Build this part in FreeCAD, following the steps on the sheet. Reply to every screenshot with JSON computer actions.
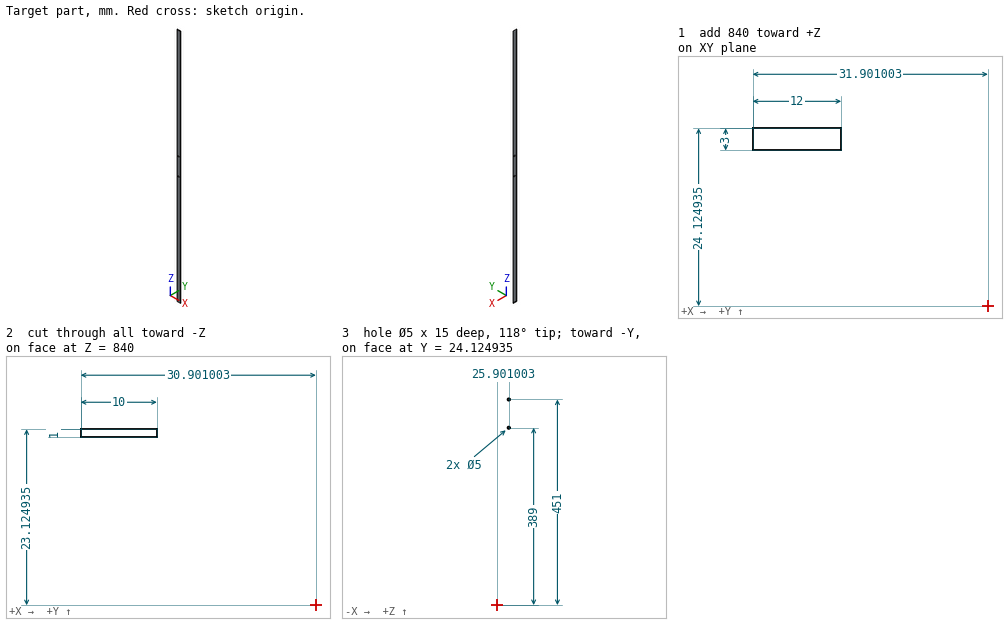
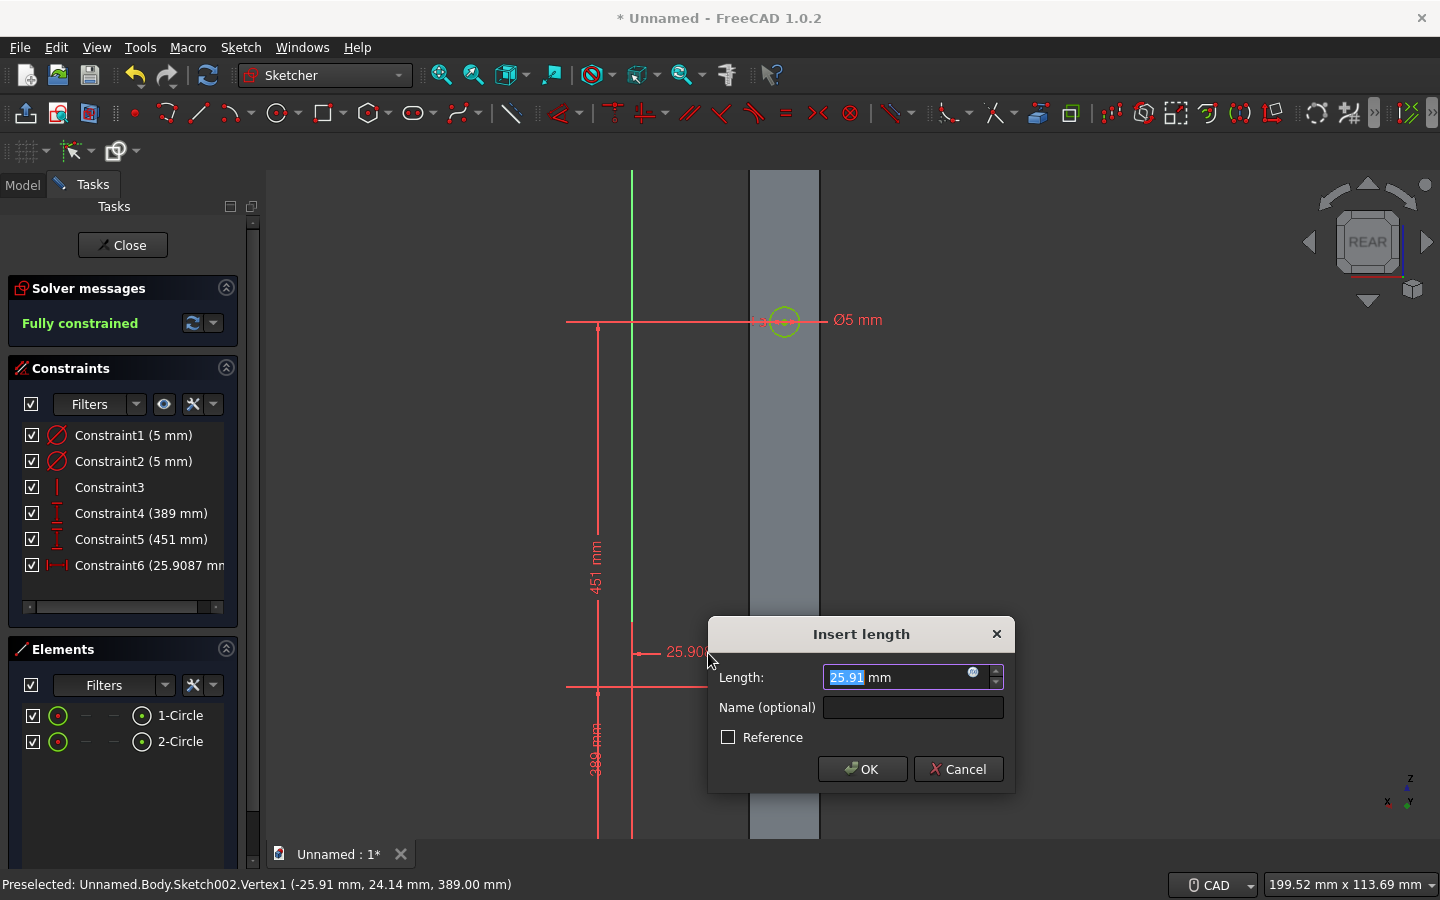
{"action": "type", "text": "25.901003"}
{"action": "key", "text": "Return"}
{"action": "key", "text": "Escape"}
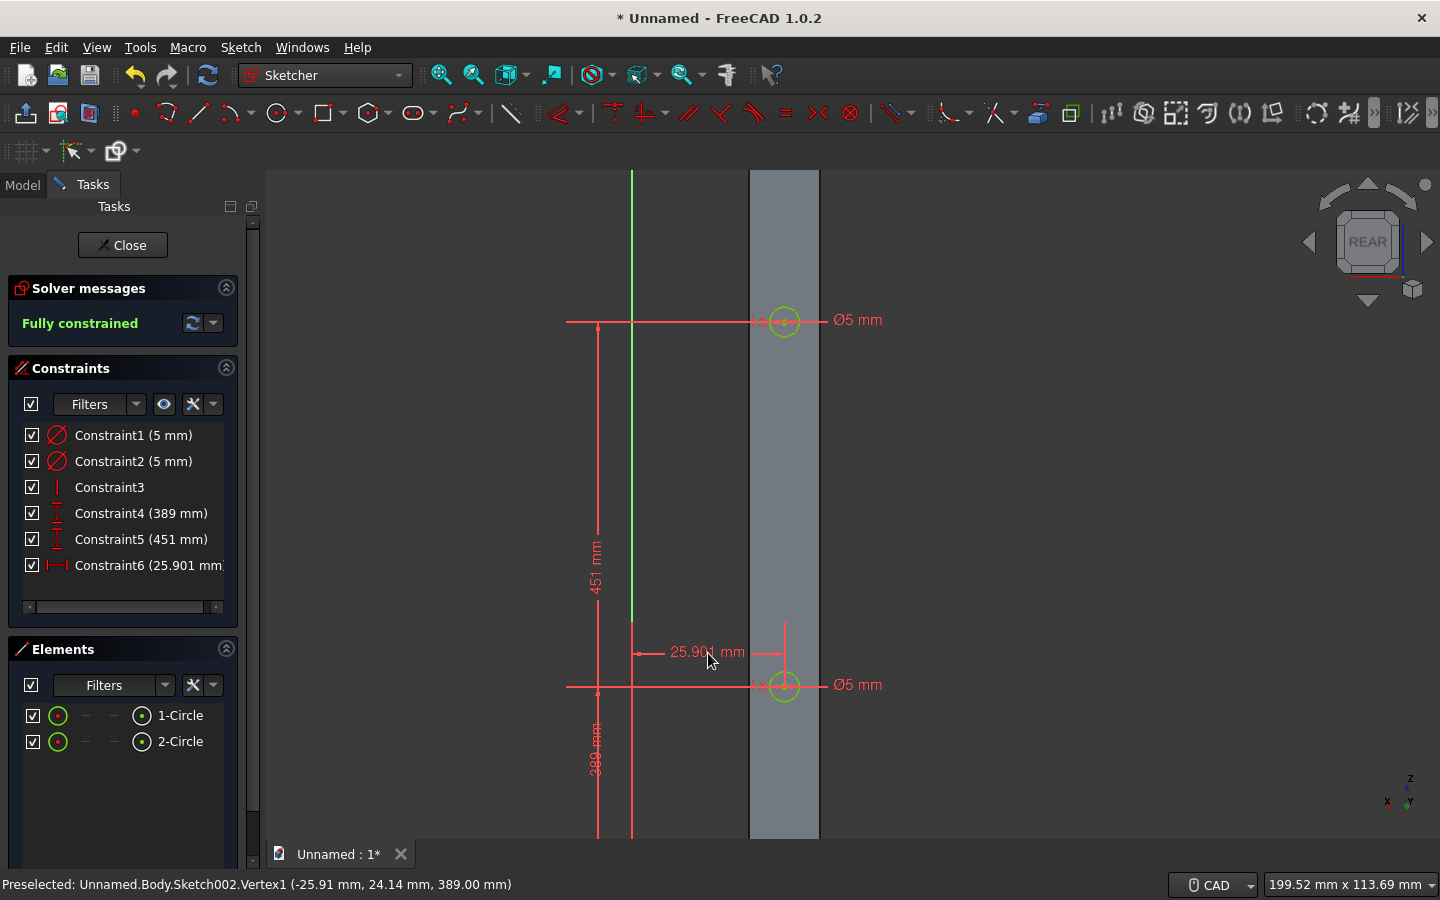
{"action": "left_click", "coordinate": [123, 245]}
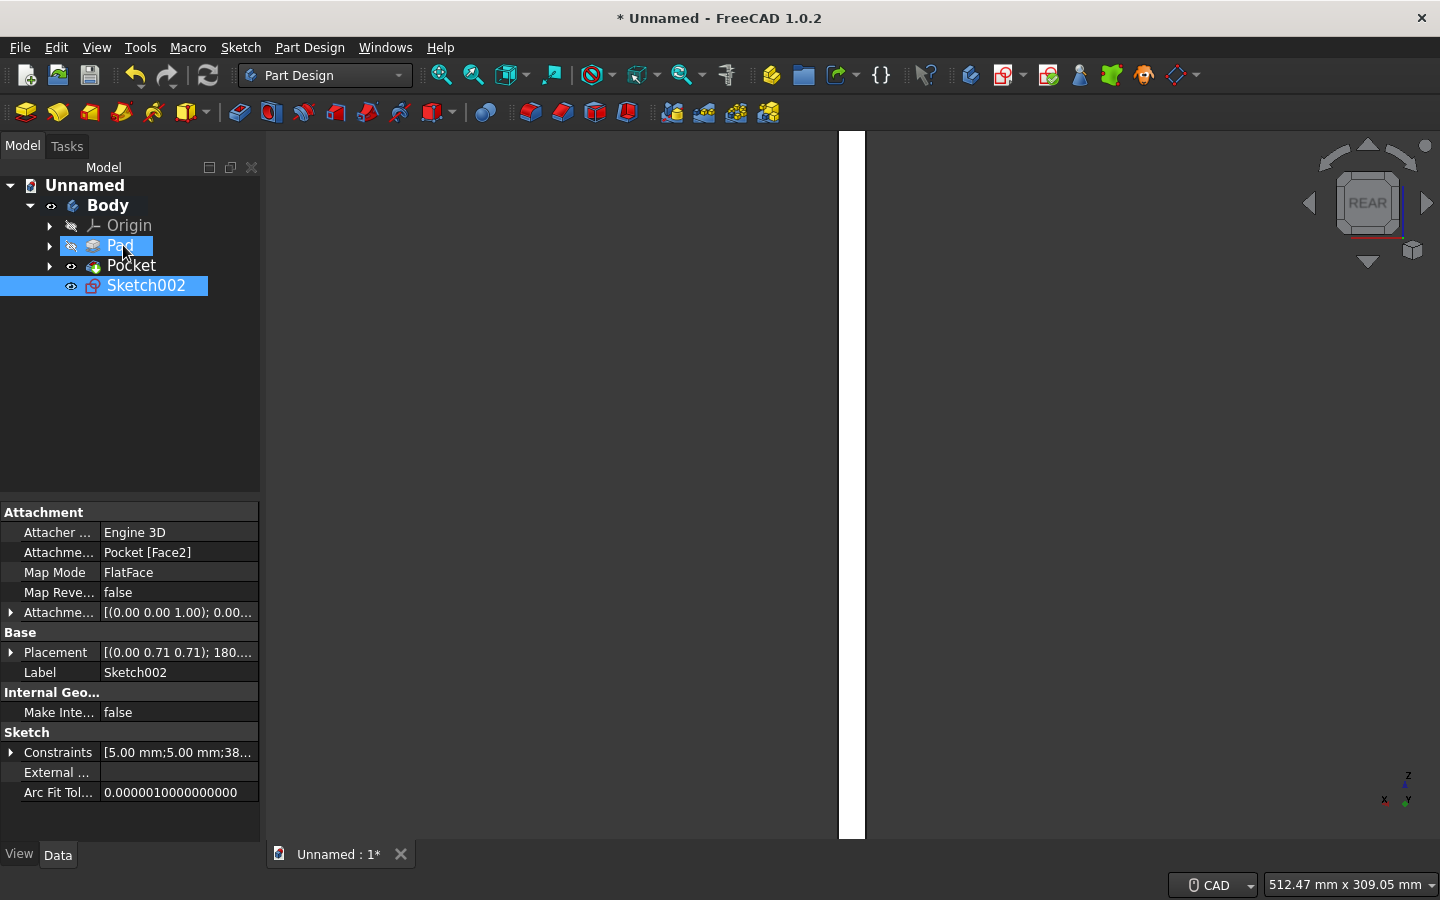
{"action": "left_click", "coordinate": [272, 112]}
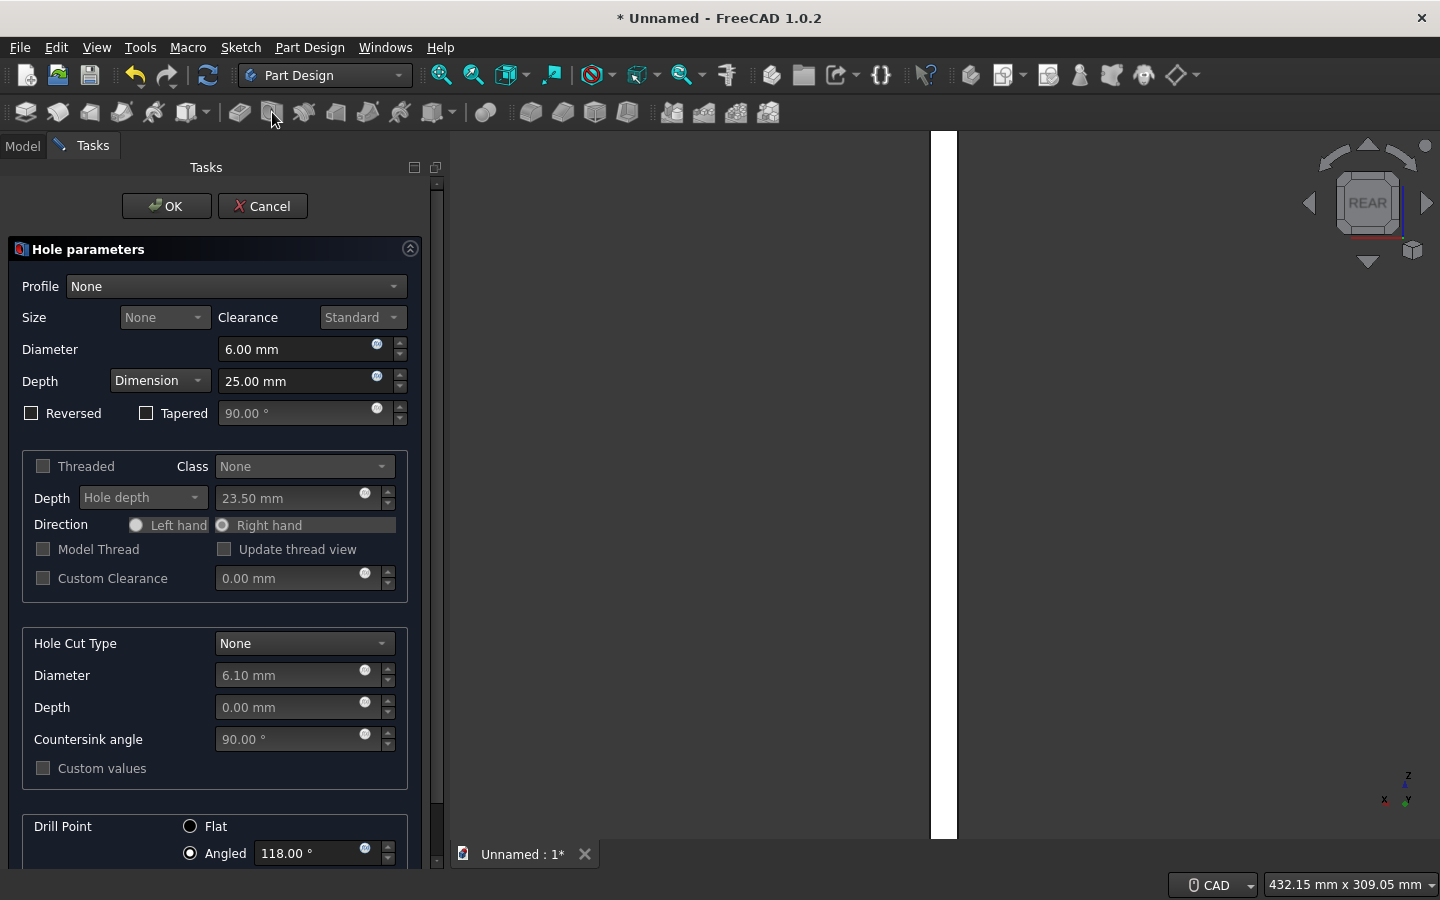
{"action": "triple_click", "coordinate": [305, 349]}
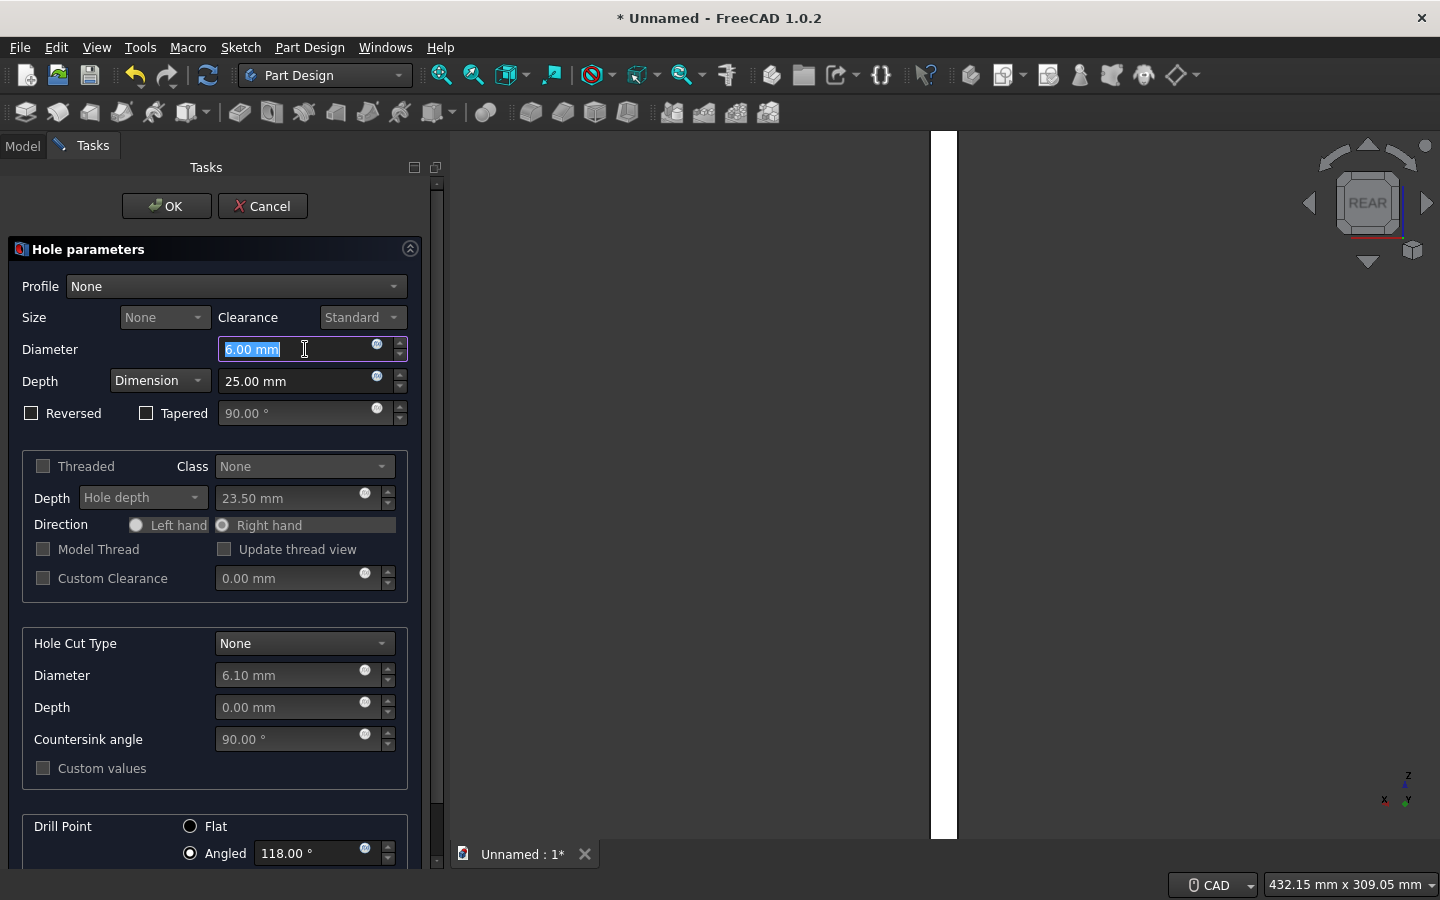
{"action": "type", "text": "5"}
{"action": "key", "text": "Tab"}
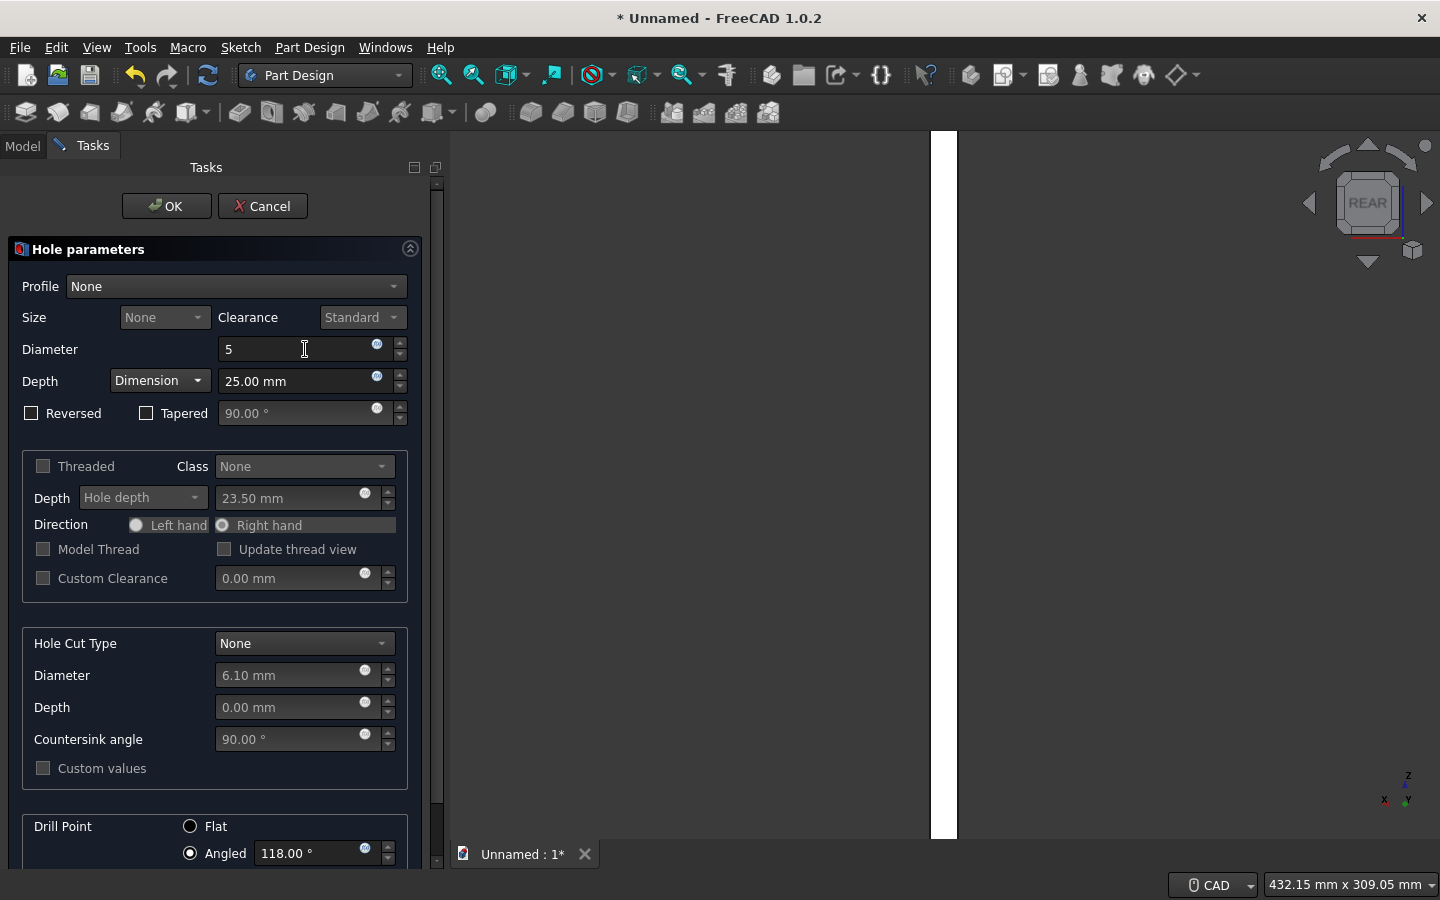
{"action": "triple_click", "coordinate": [305, 381]}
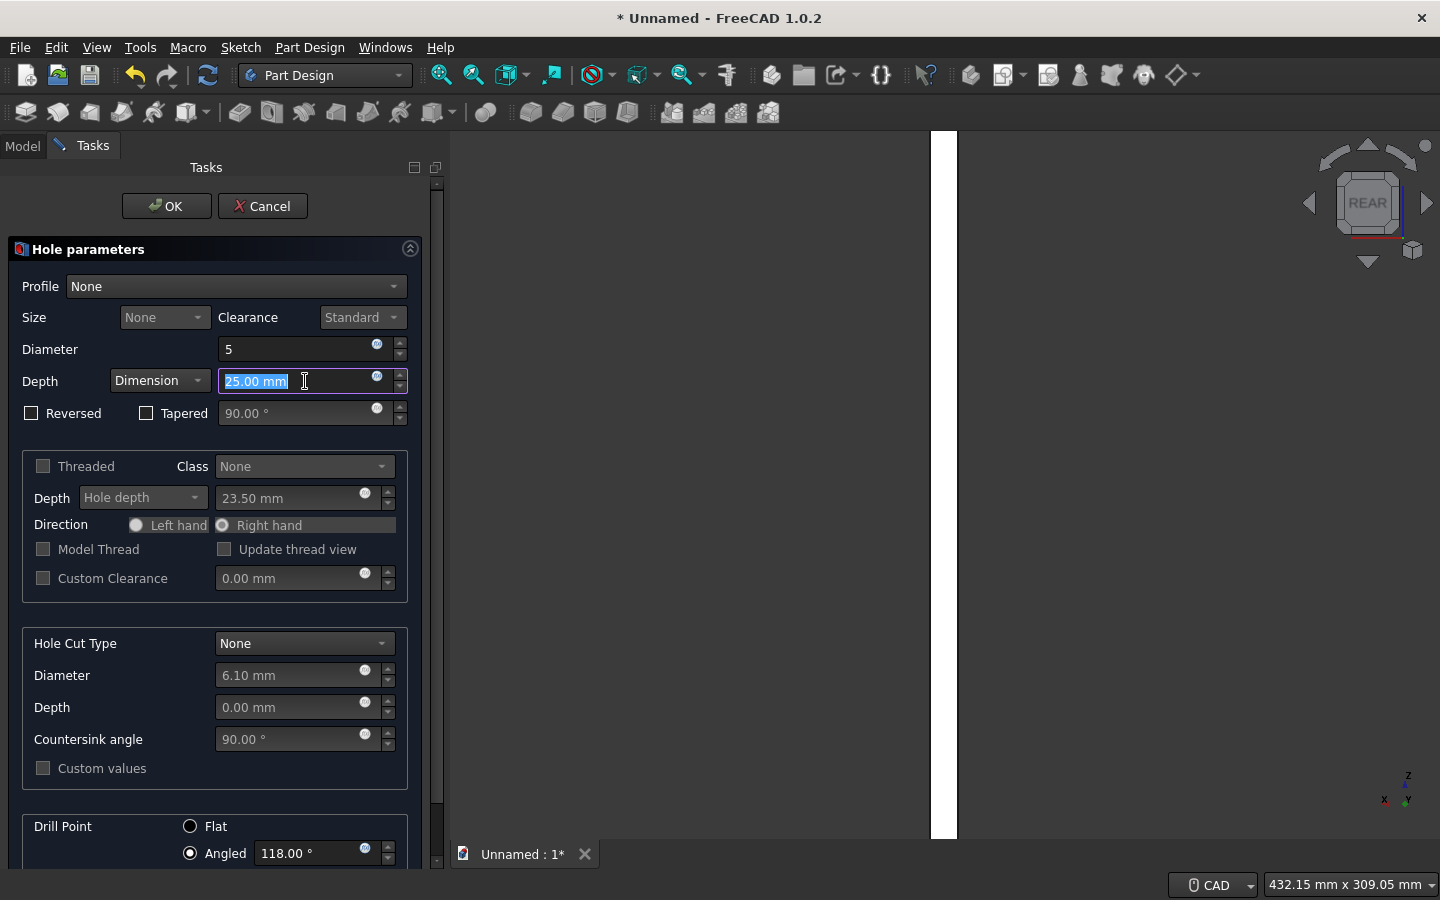
{"action": "type", "text": "15"}
{"action": "key", "text": "Tab"}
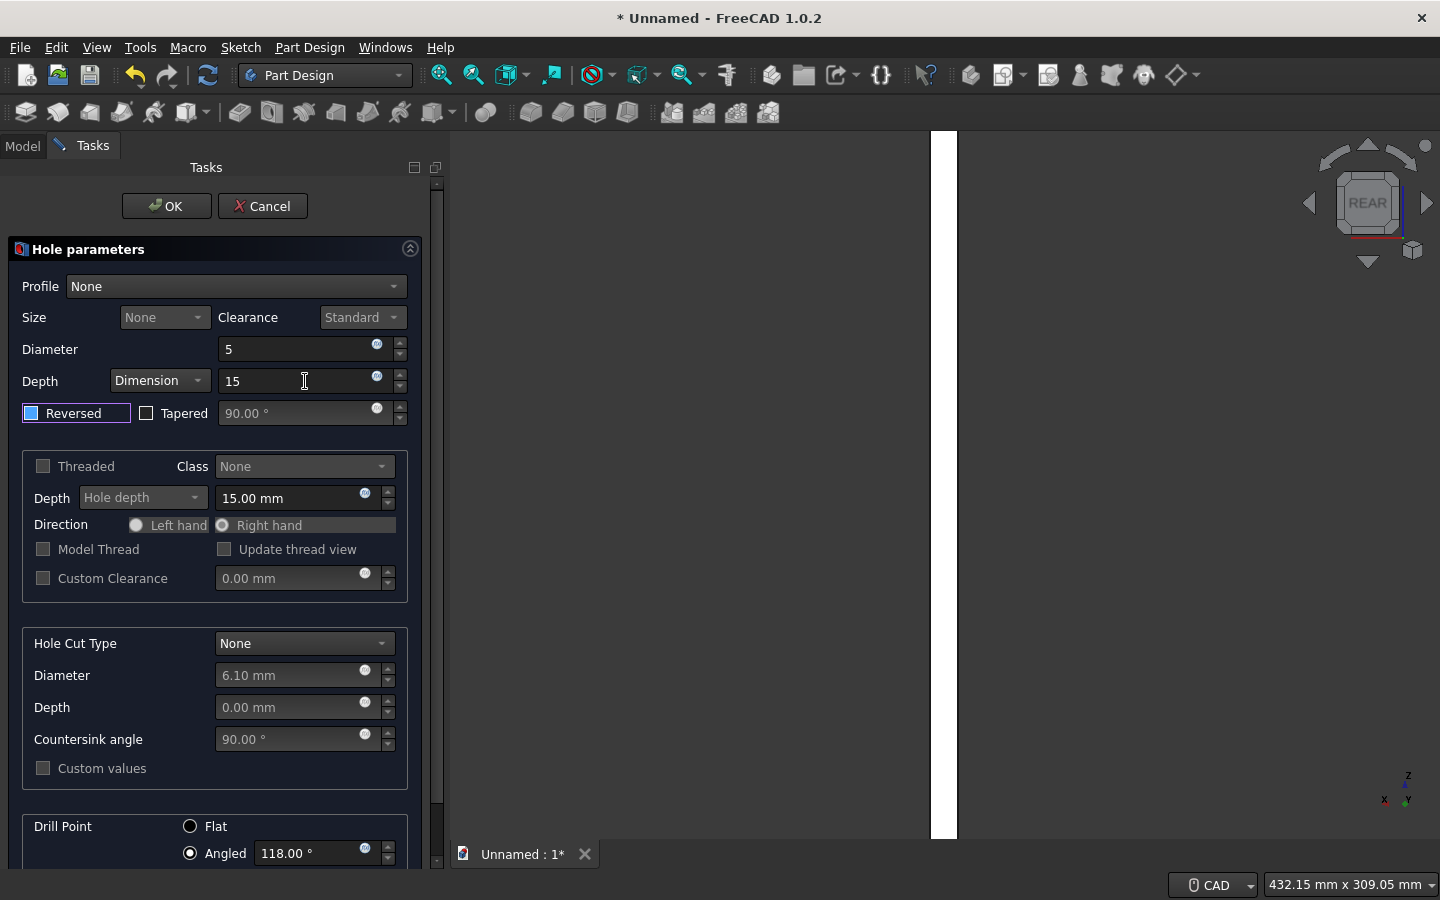
{"action": "left_click", "coordinate": [167, 206]}